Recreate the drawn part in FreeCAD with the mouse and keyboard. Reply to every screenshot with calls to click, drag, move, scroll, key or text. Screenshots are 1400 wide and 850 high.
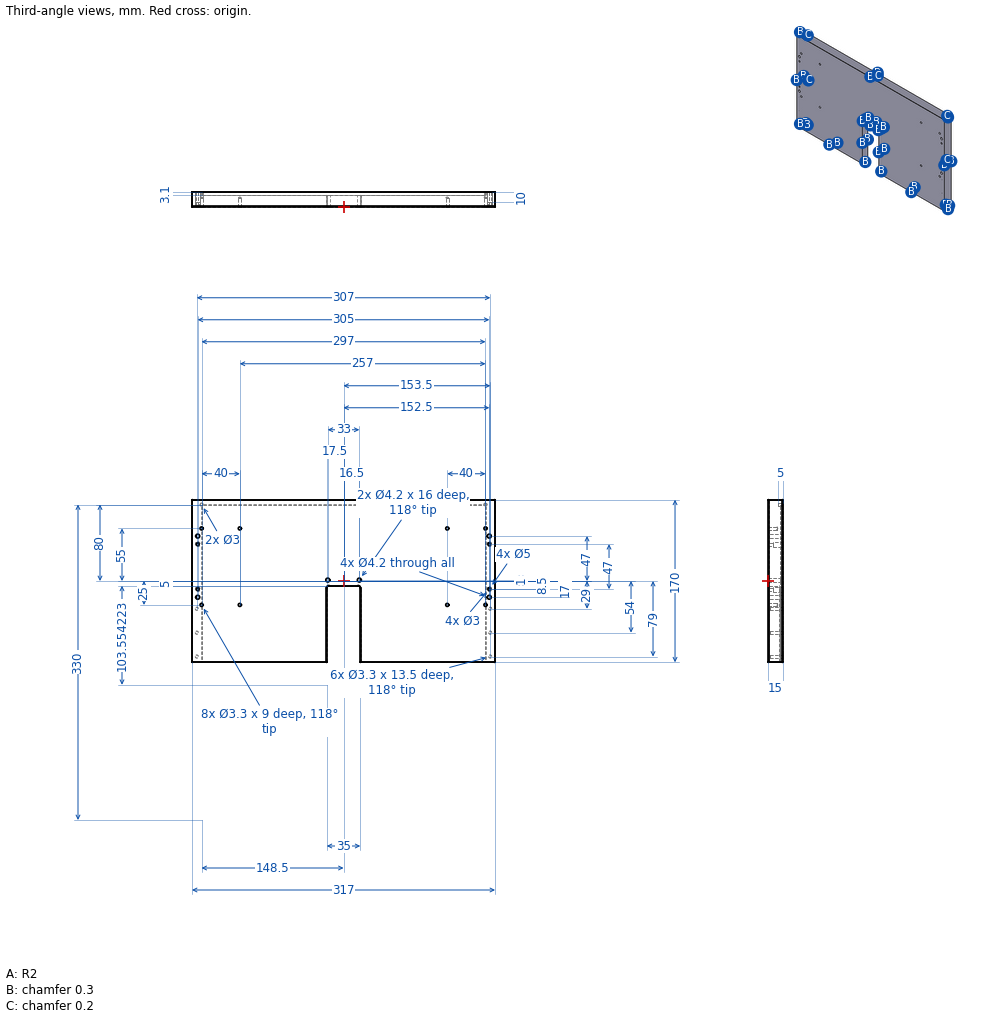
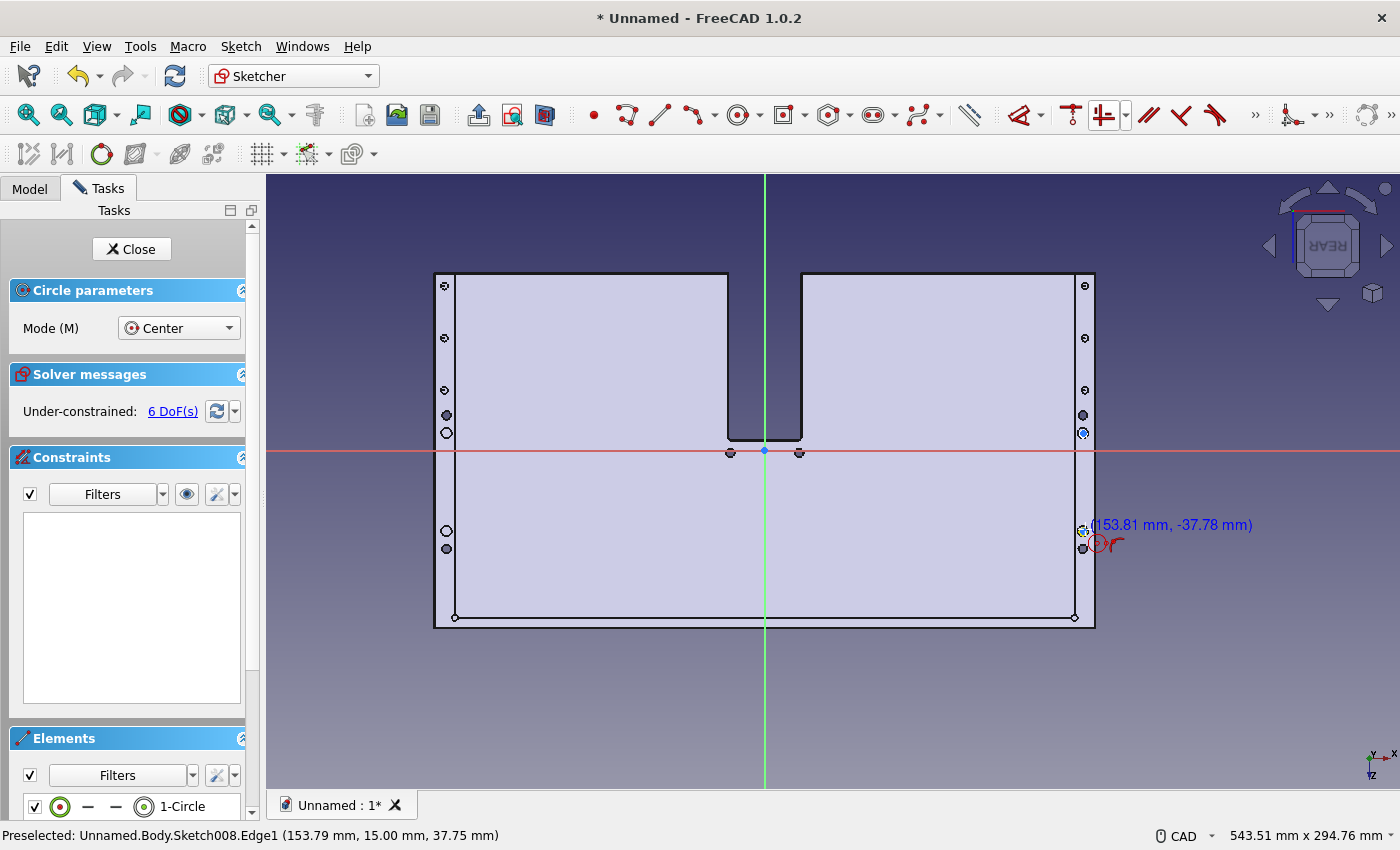
scroll(447, 433, up, 10)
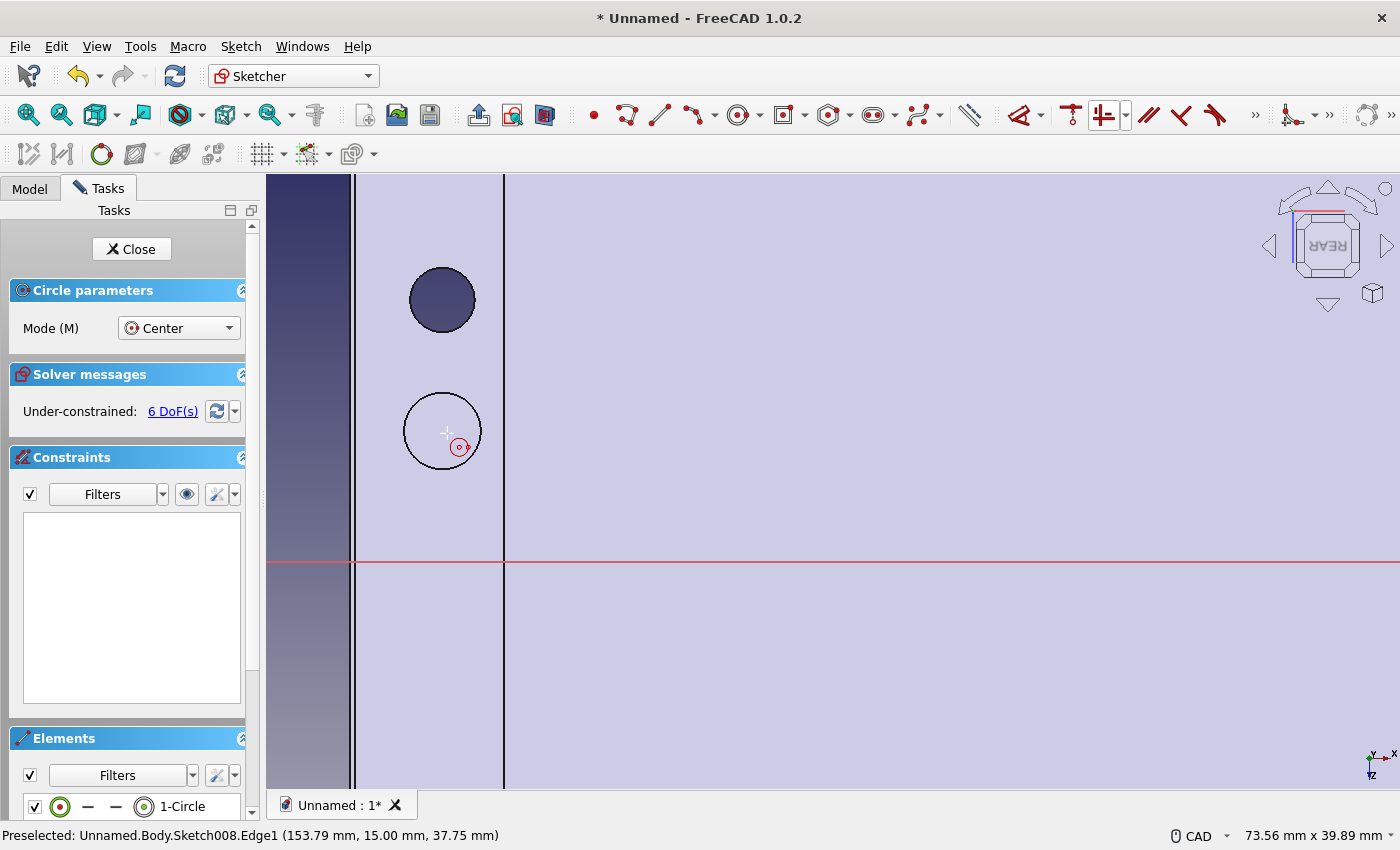
scroll(447, 433, down, 10)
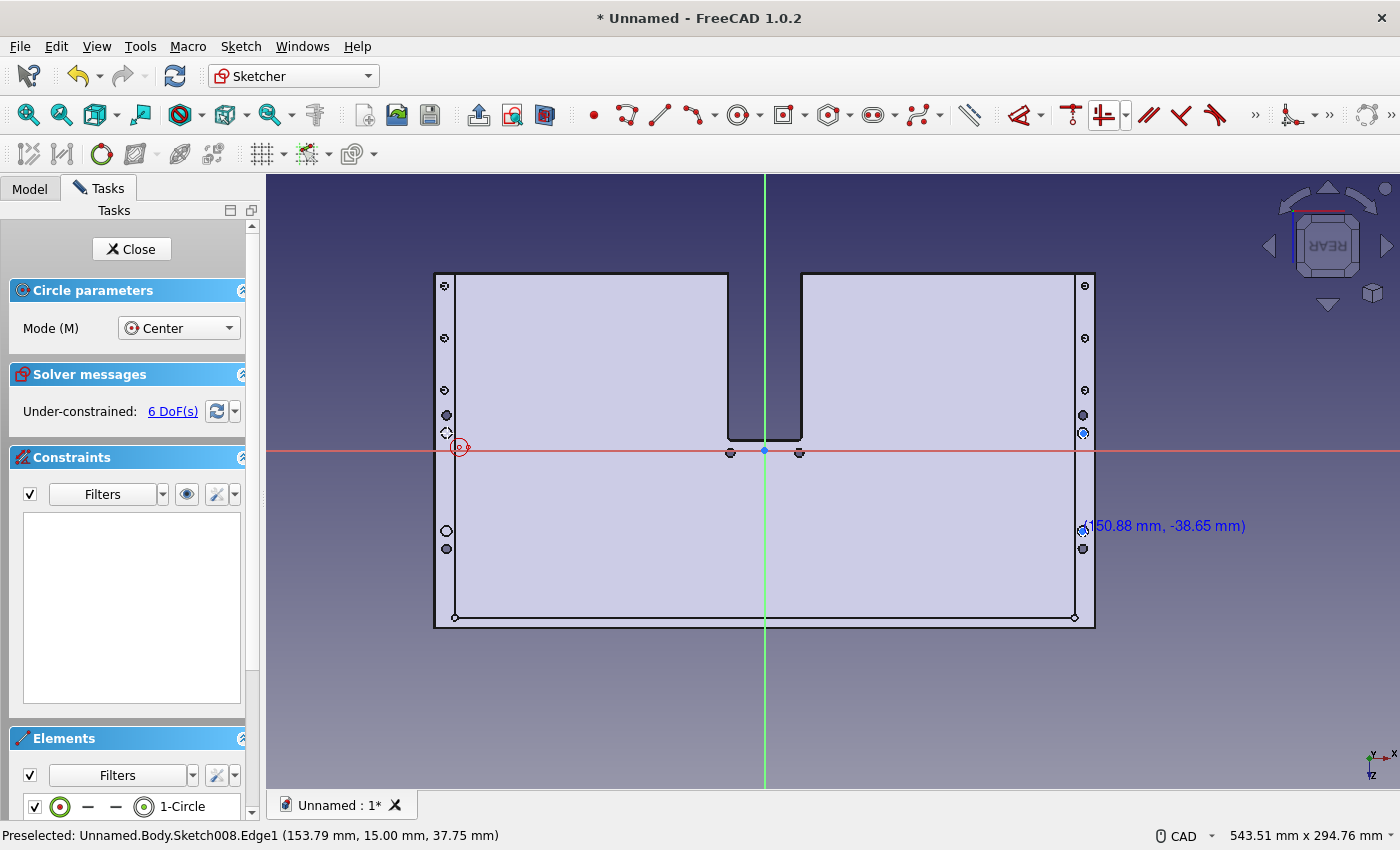
click(447, 433)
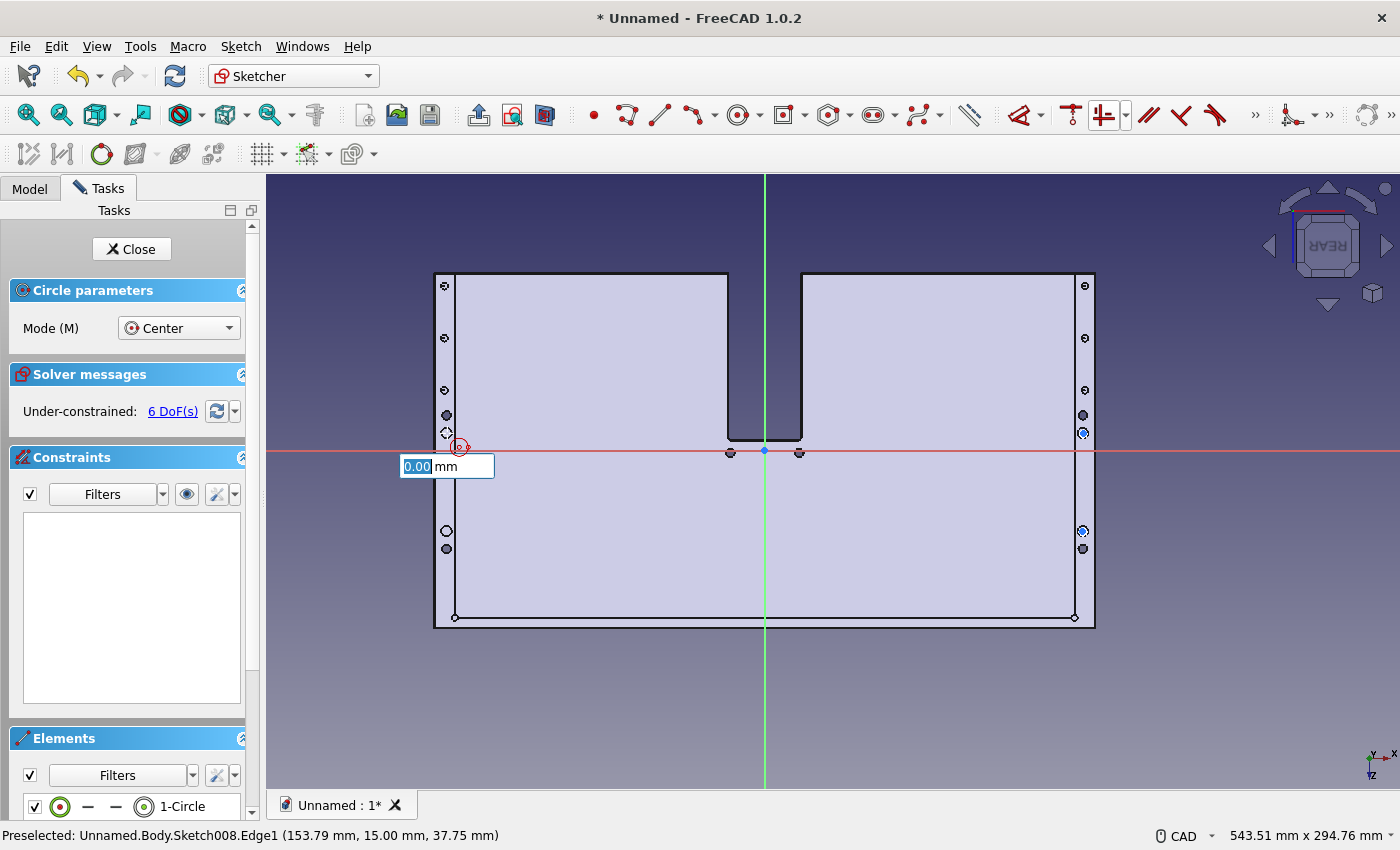
scroll(449, 431, up, 9)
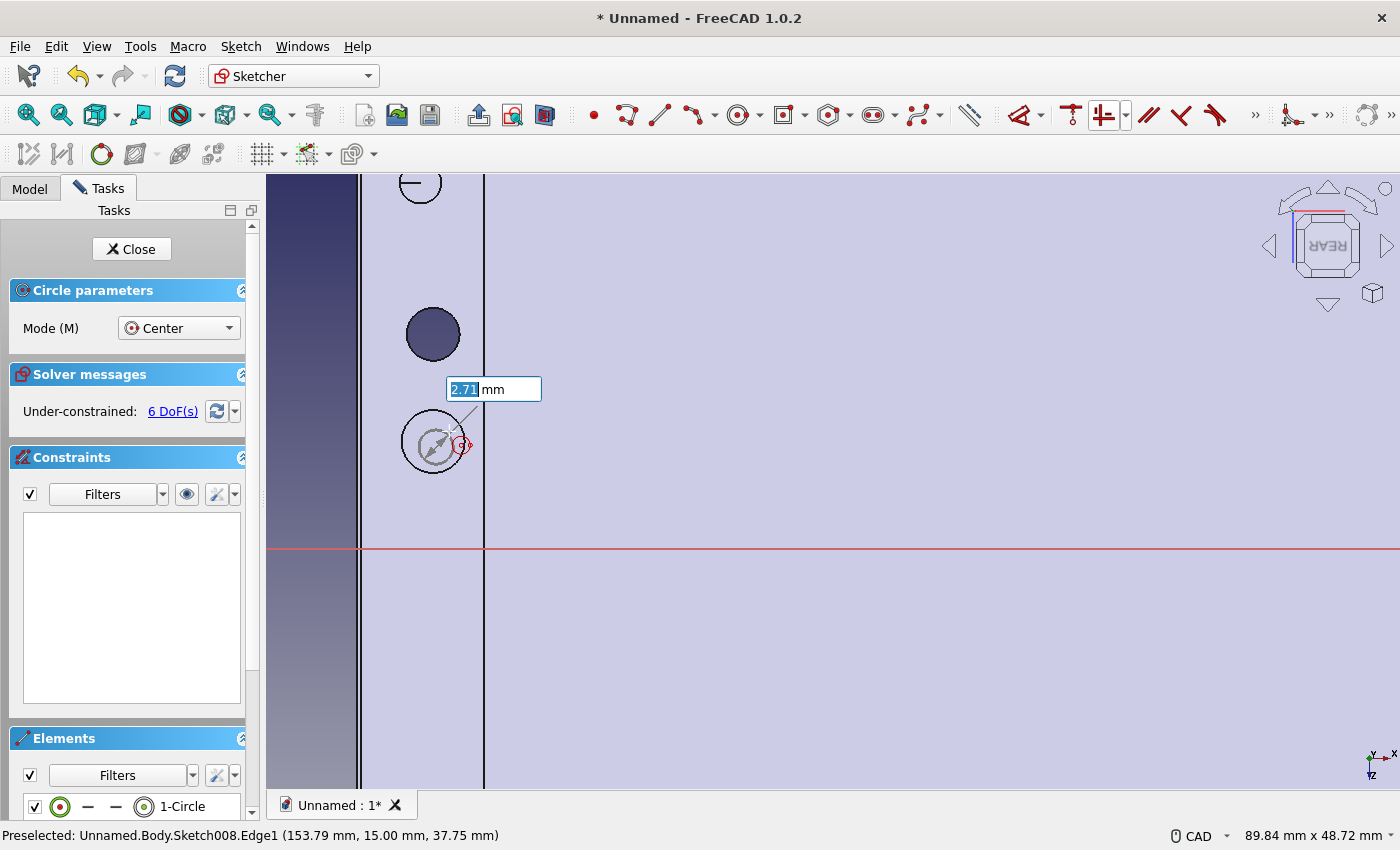
click(447, 428)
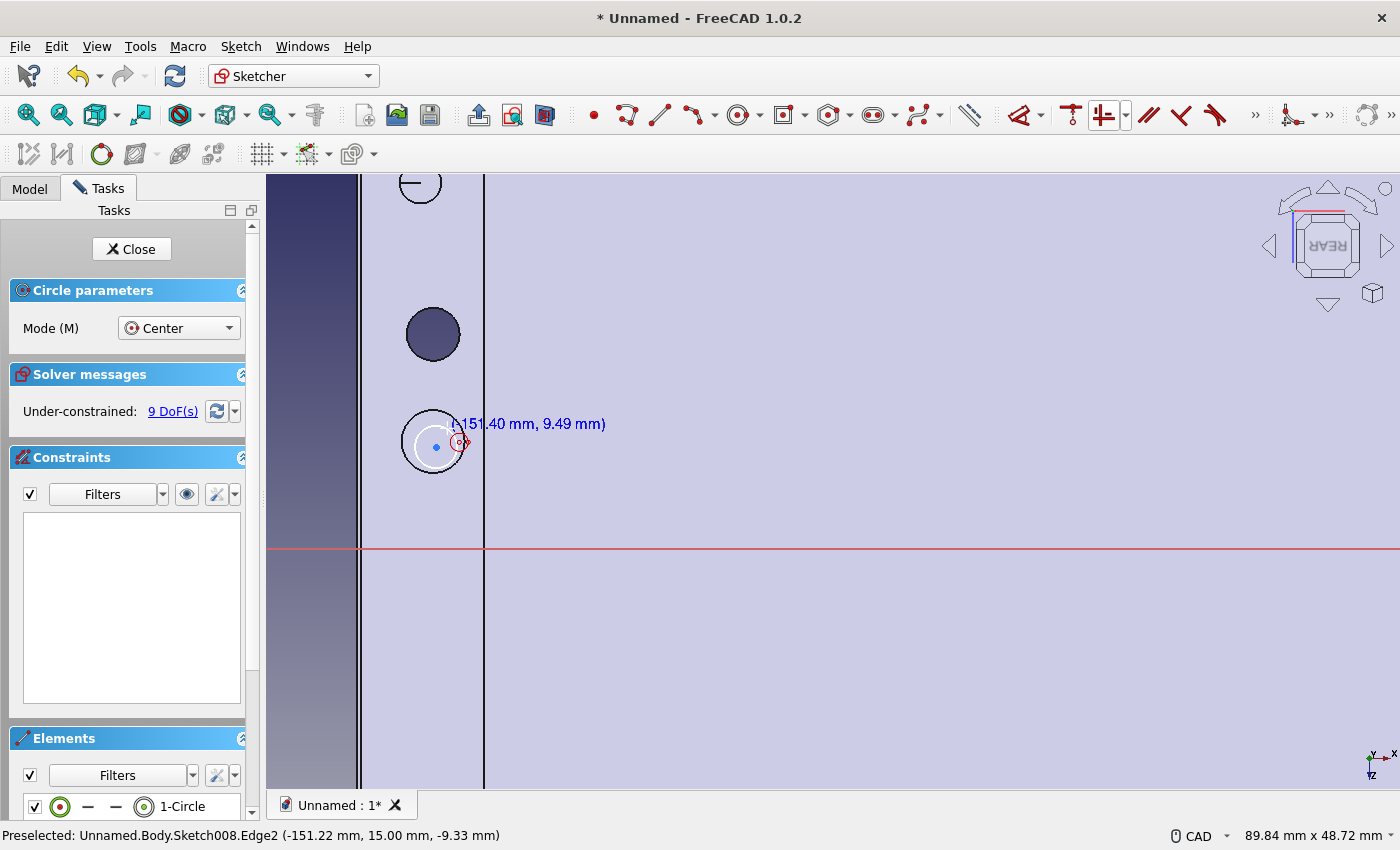
scroll(449, 431, down, 9)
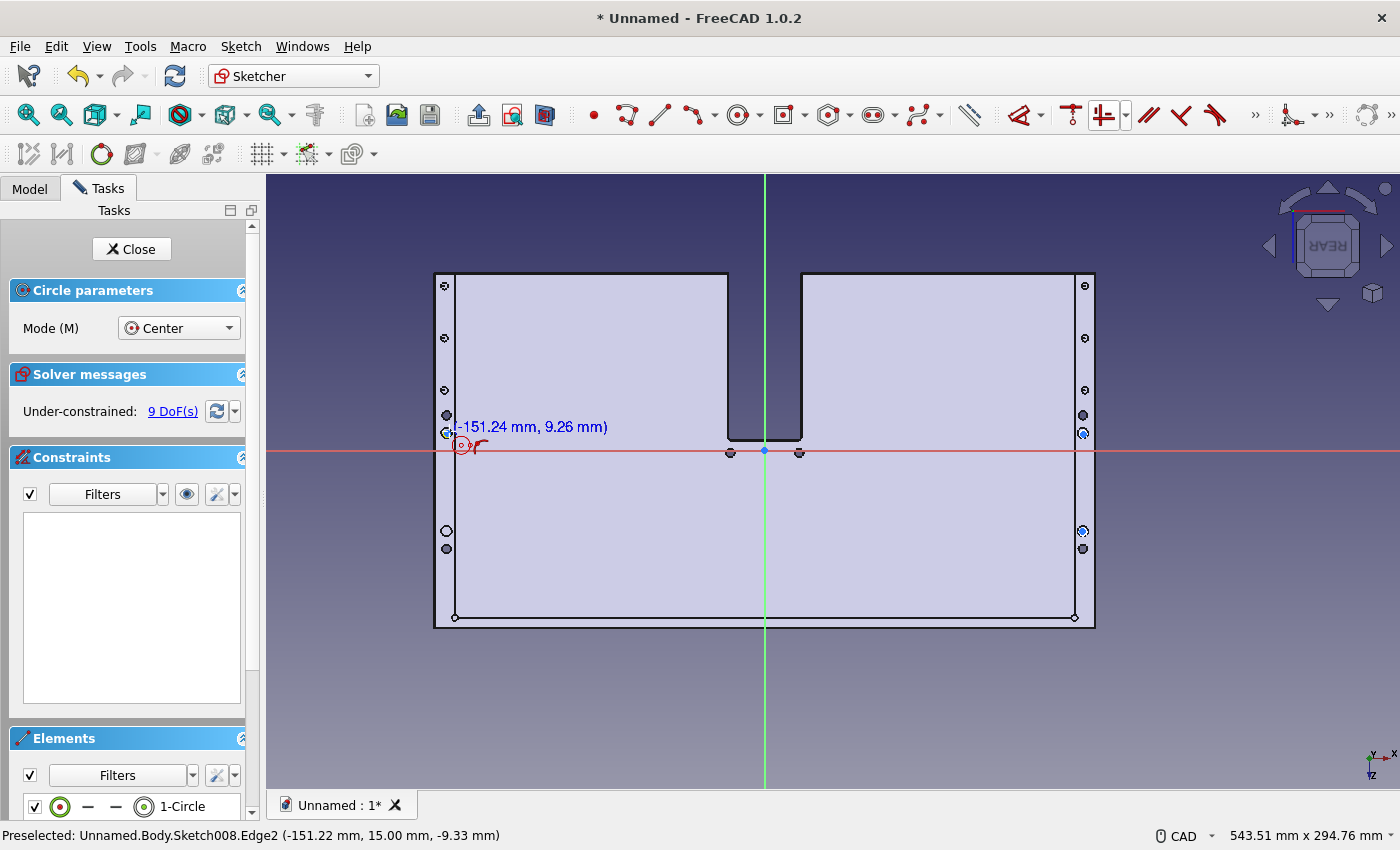
scroll(447, 531, up, 10)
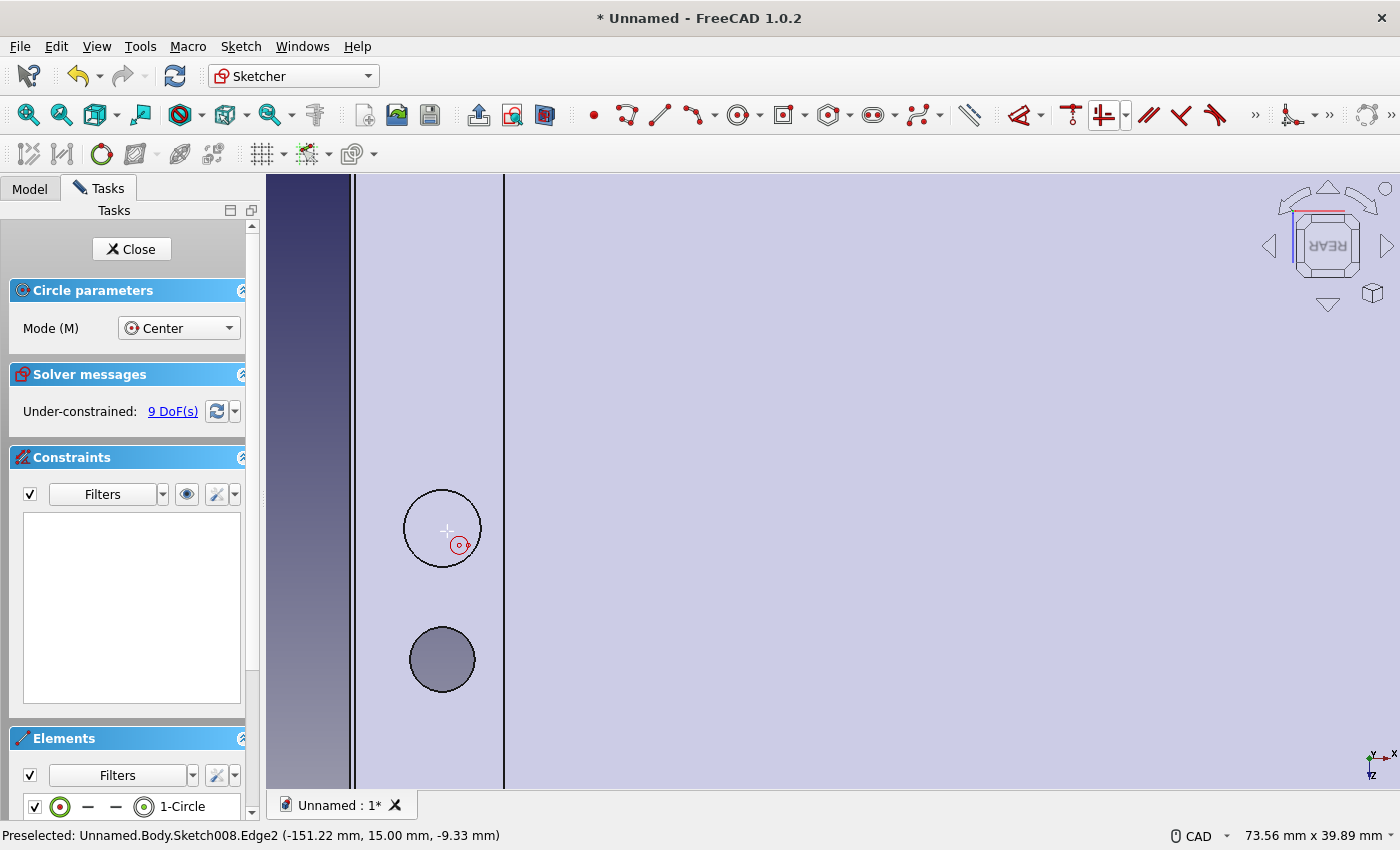
scroll(447, 531, down, 10)